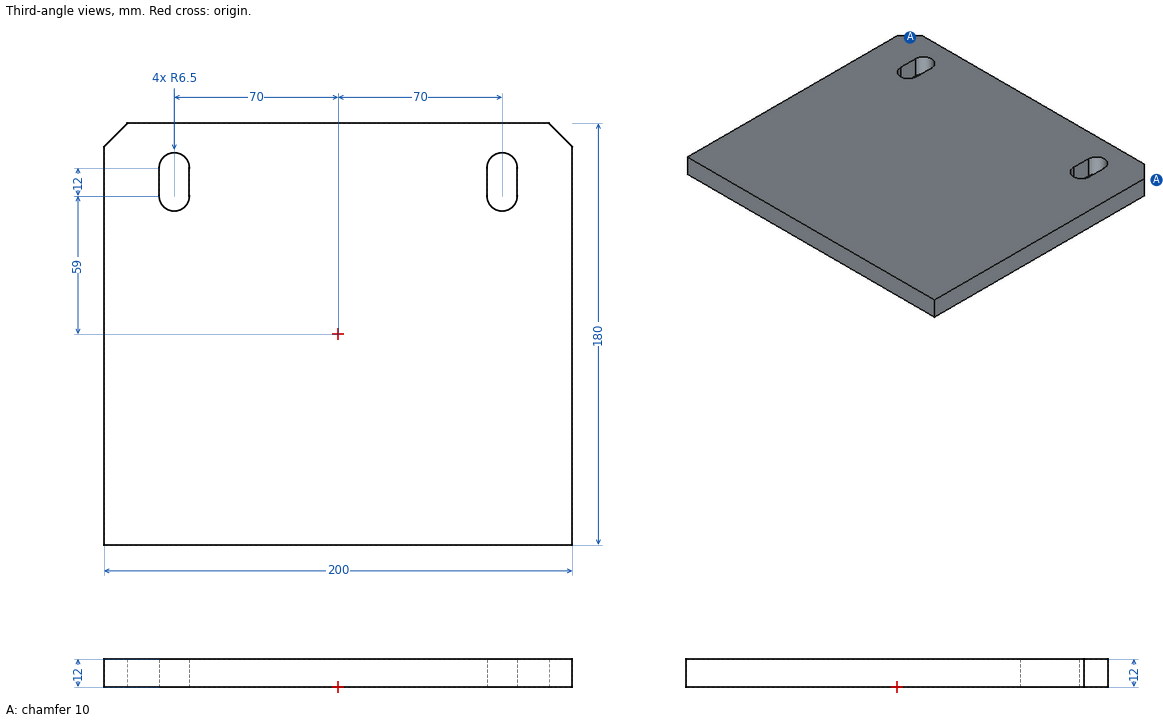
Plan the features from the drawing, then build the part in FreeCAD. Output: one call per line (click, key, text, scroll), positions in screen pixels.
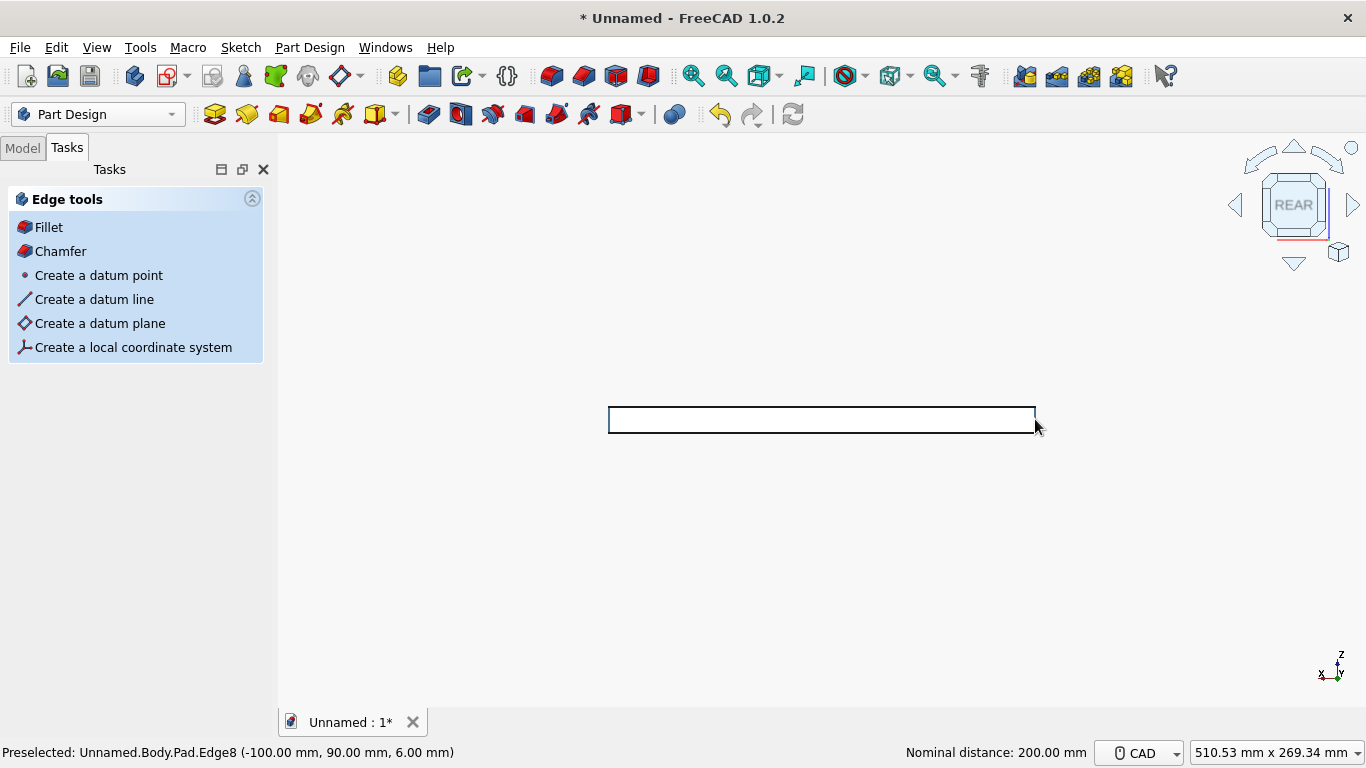
click(584, 76)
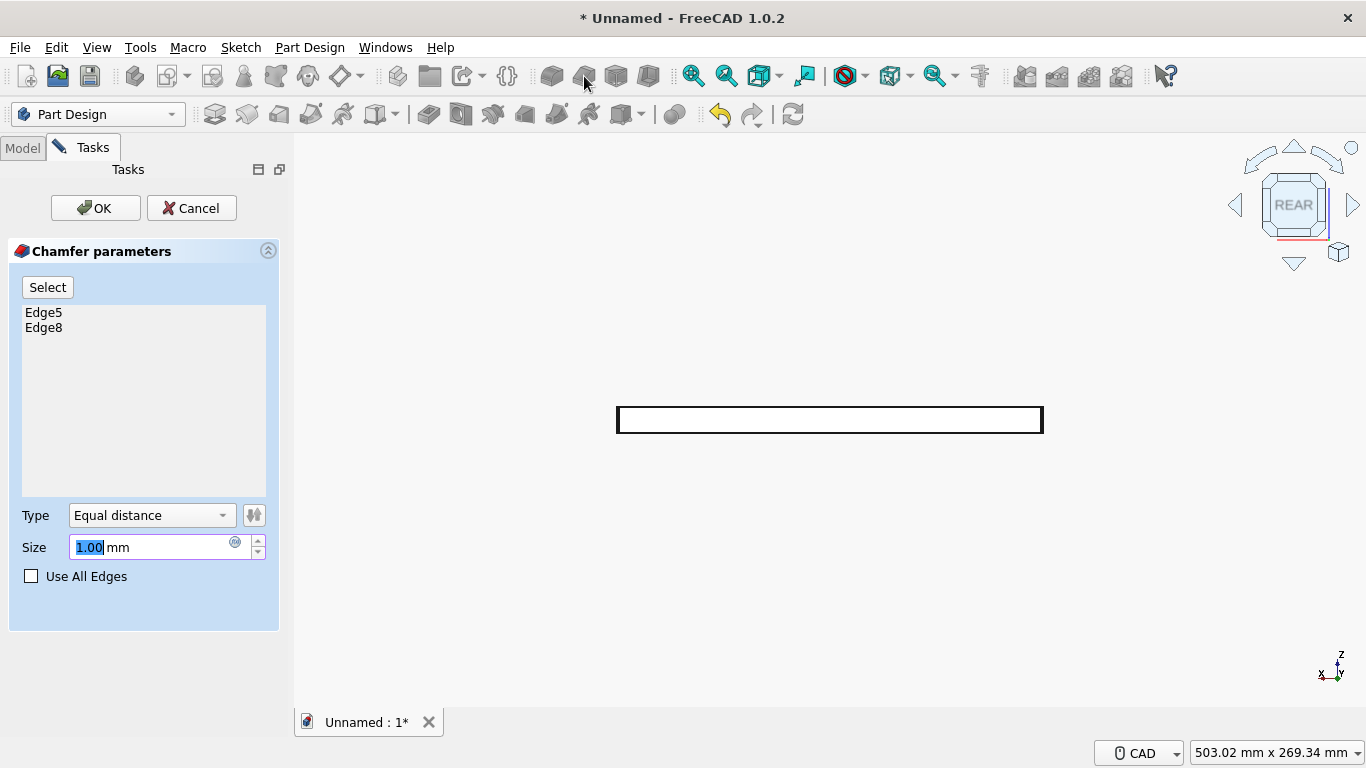
text(10)
key(Tab)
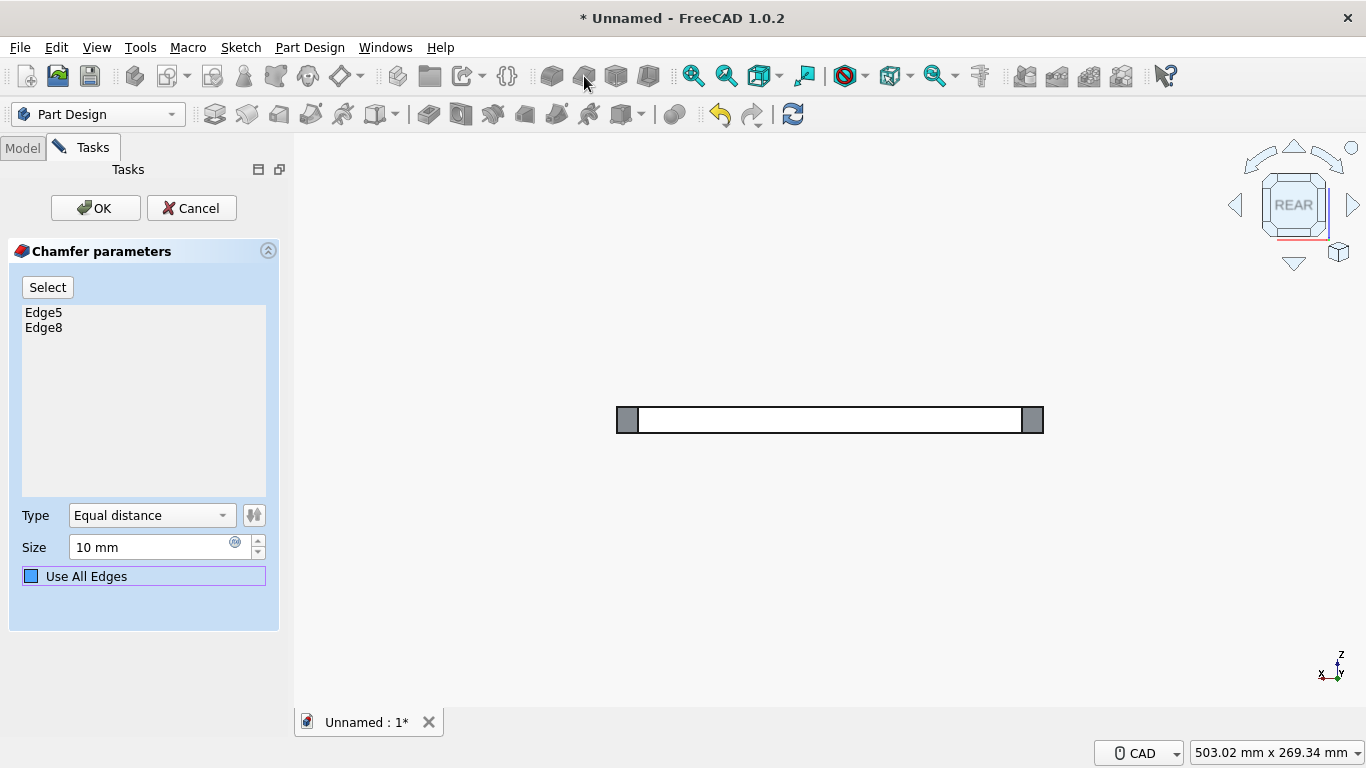
click(96, 208)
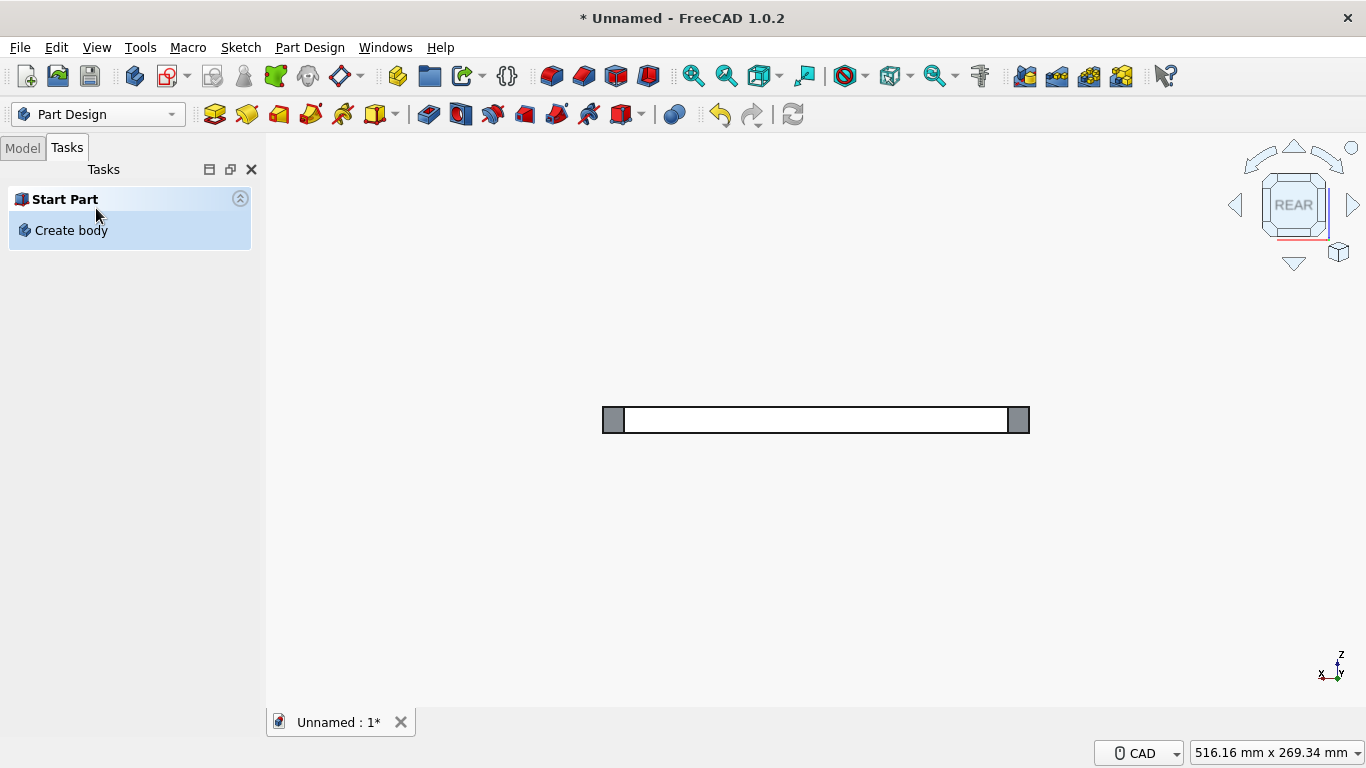
click(694, 76)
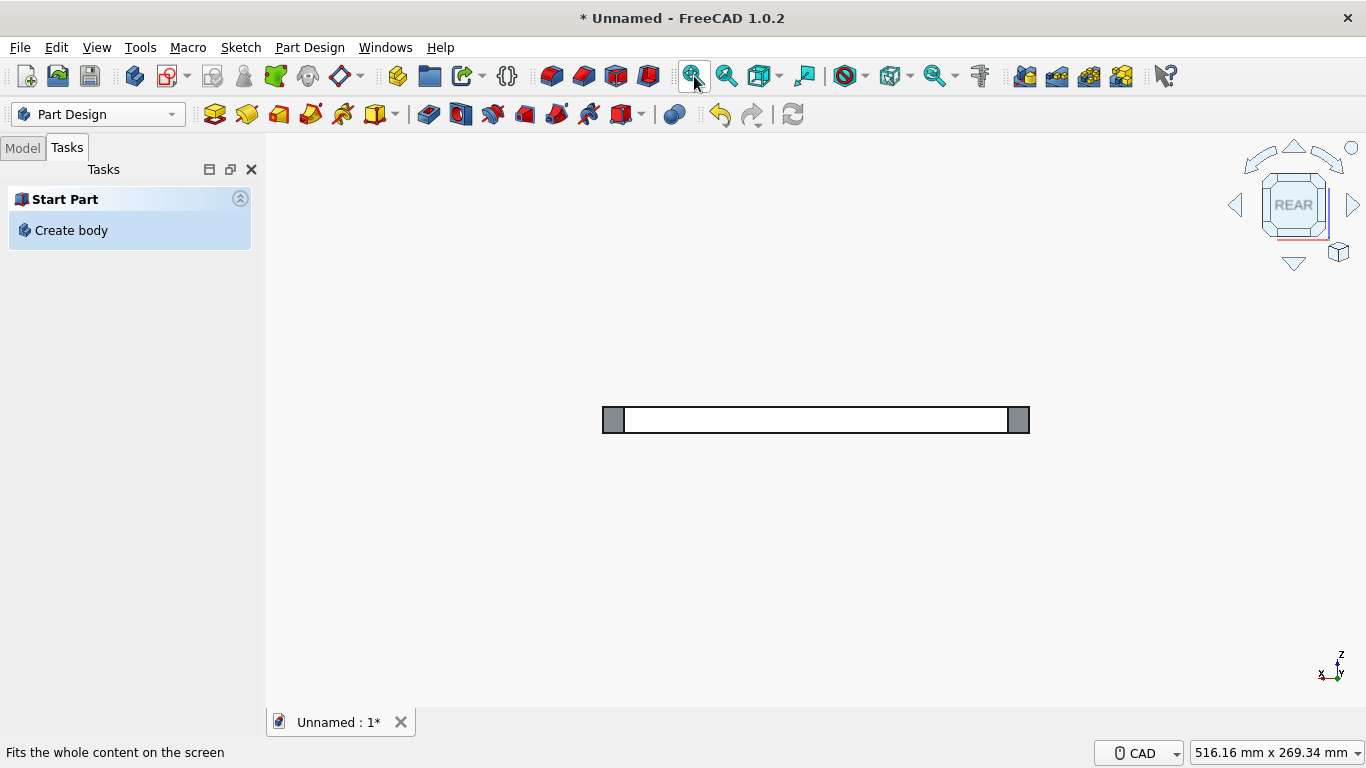
key(0)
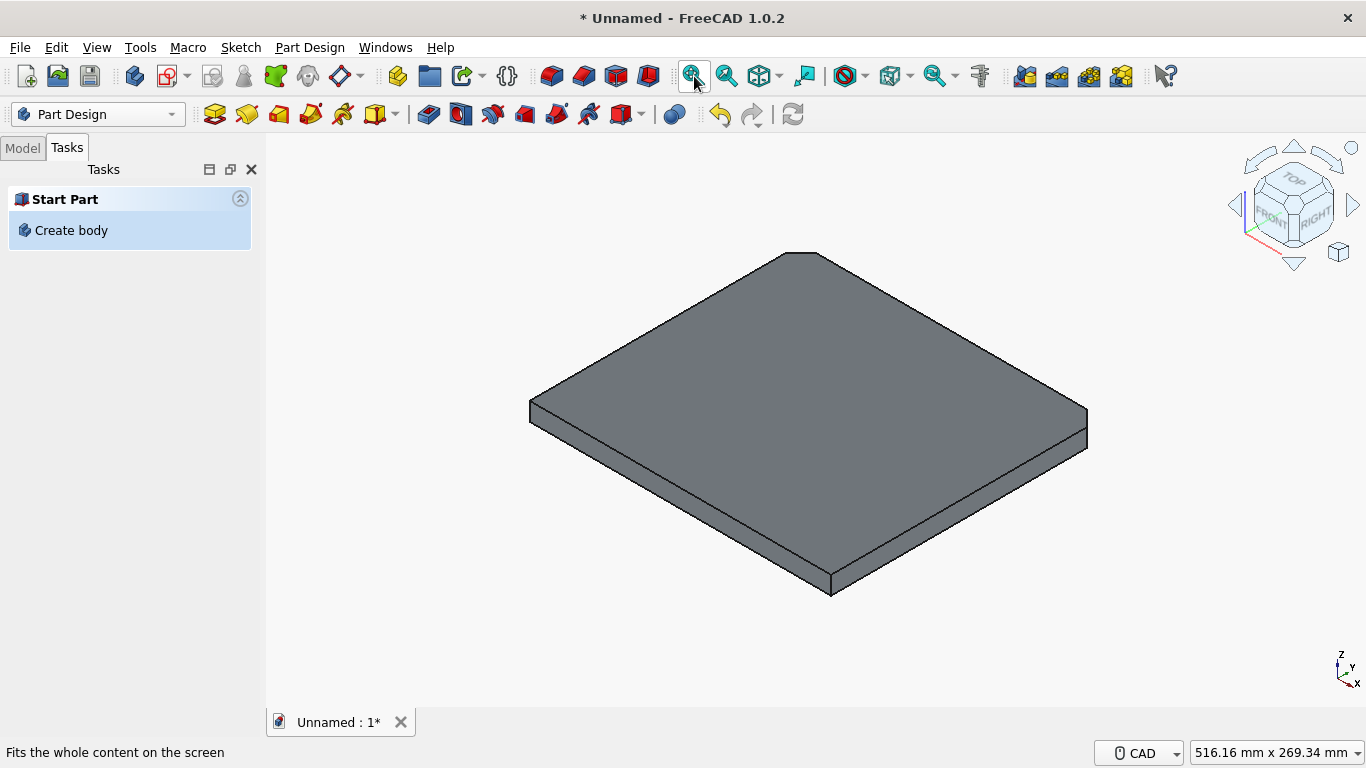
click(816, 409)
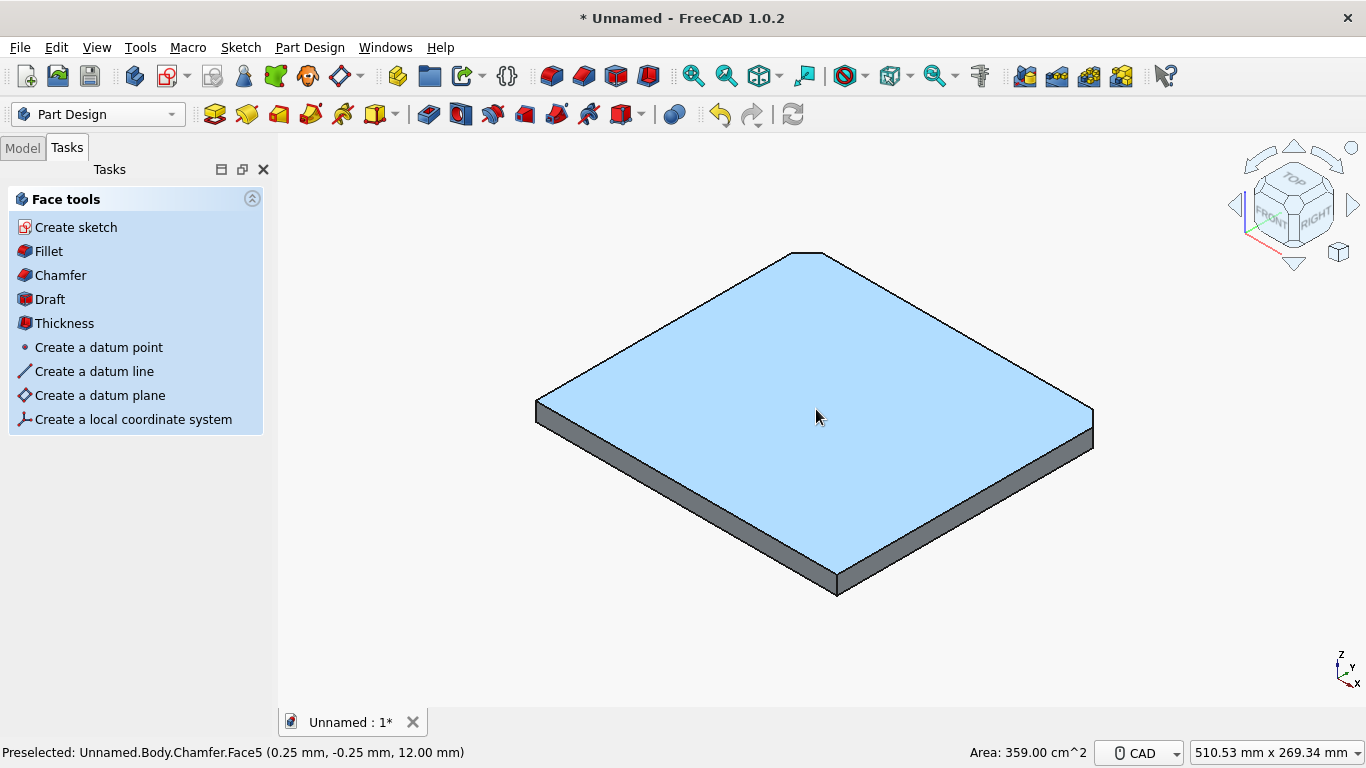
click(168, 76)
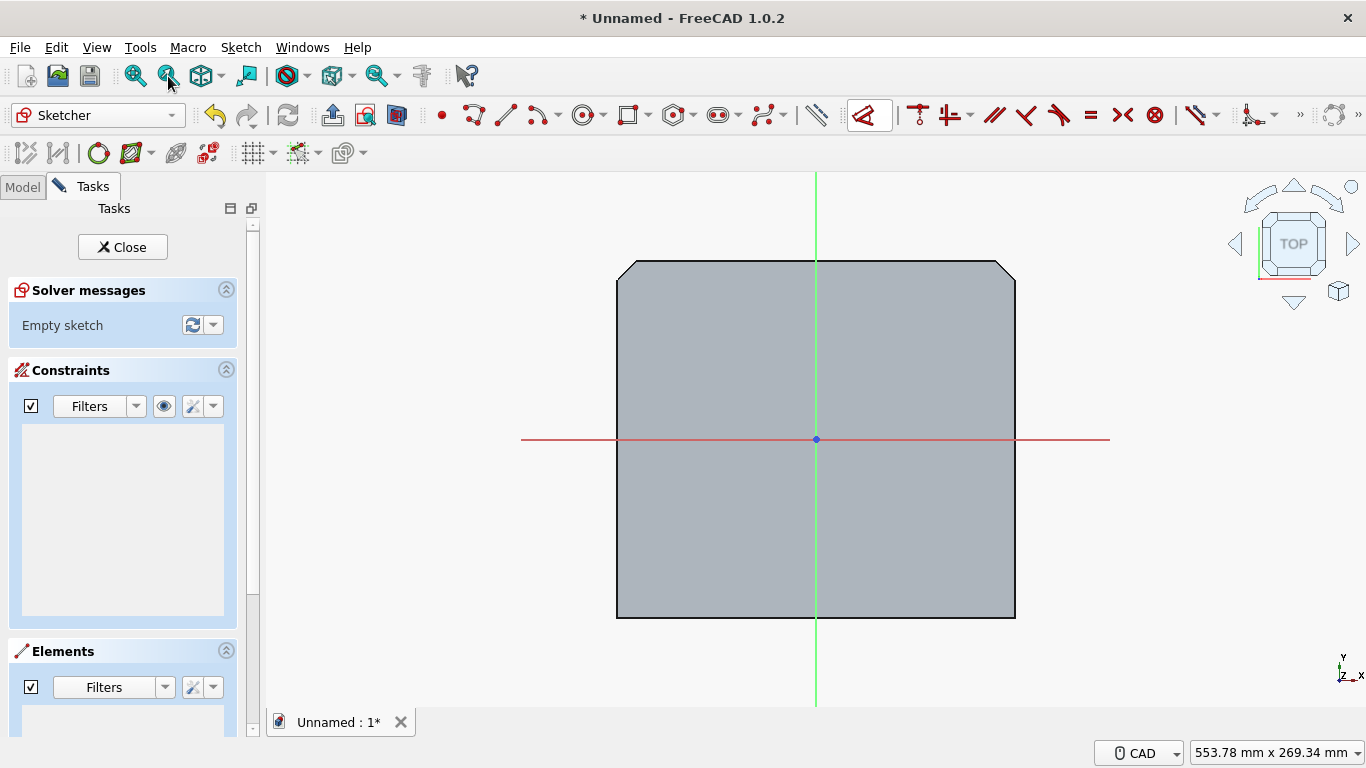
scroll(872, 300, up, 4)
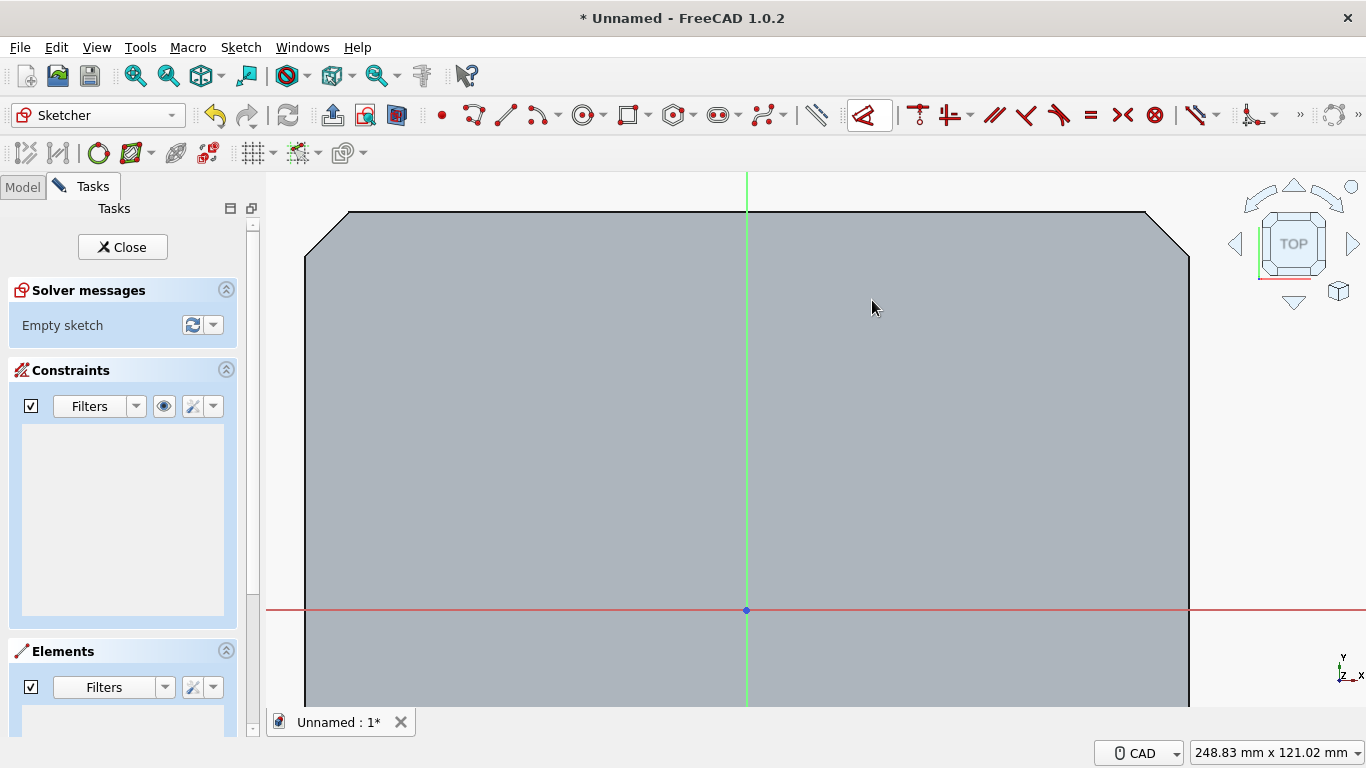
key(g)
key(s)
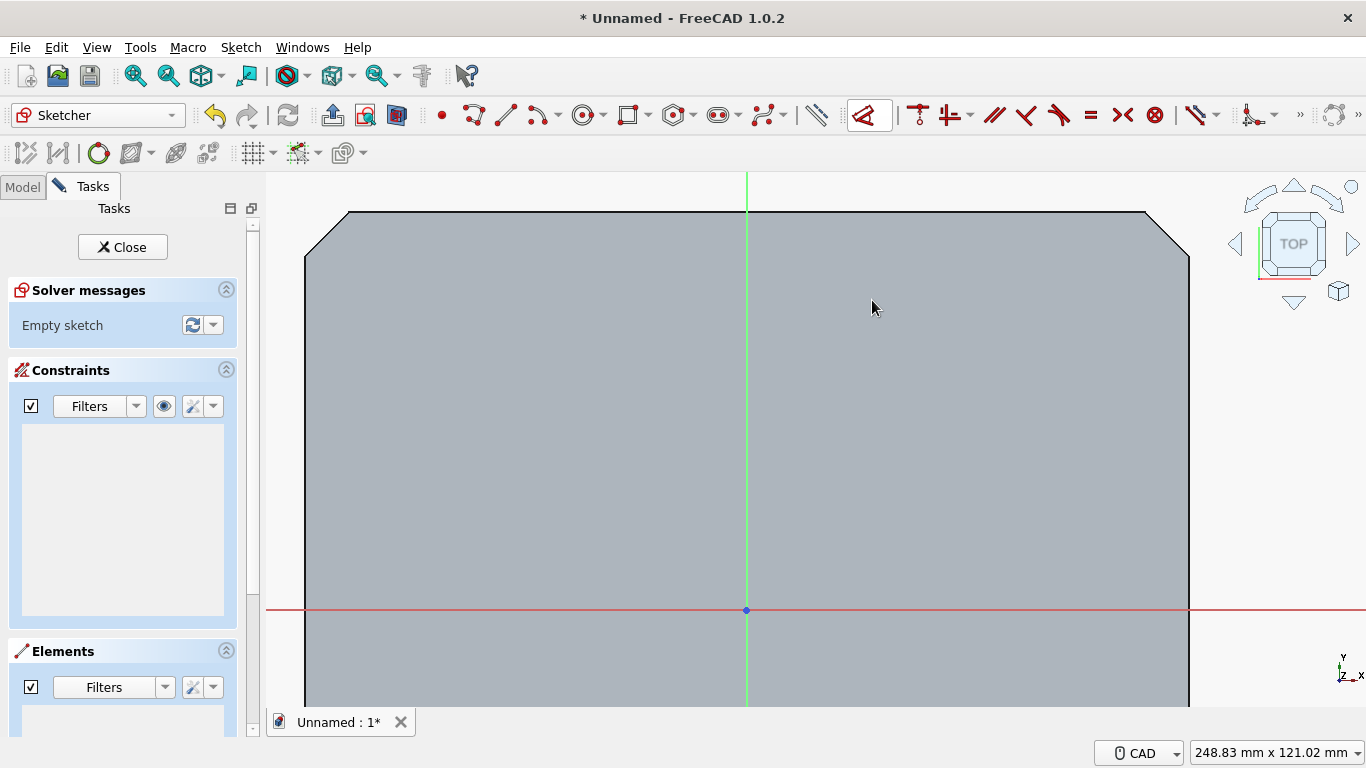
click(437, 349)